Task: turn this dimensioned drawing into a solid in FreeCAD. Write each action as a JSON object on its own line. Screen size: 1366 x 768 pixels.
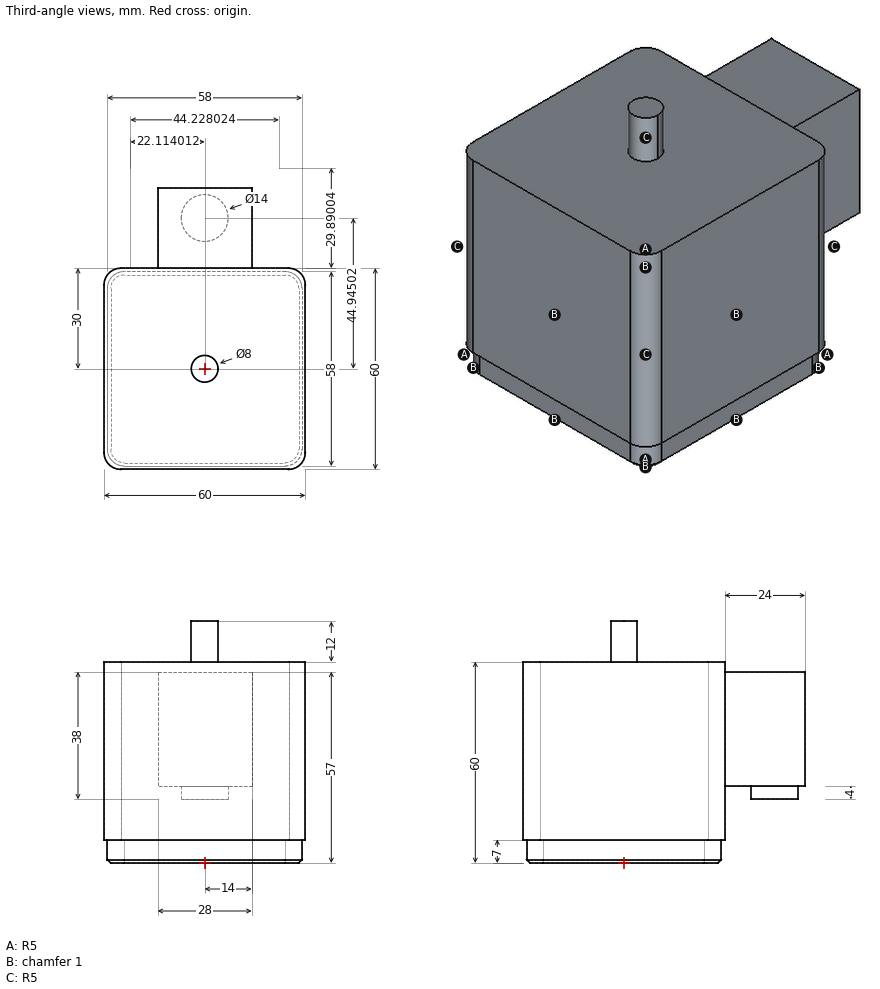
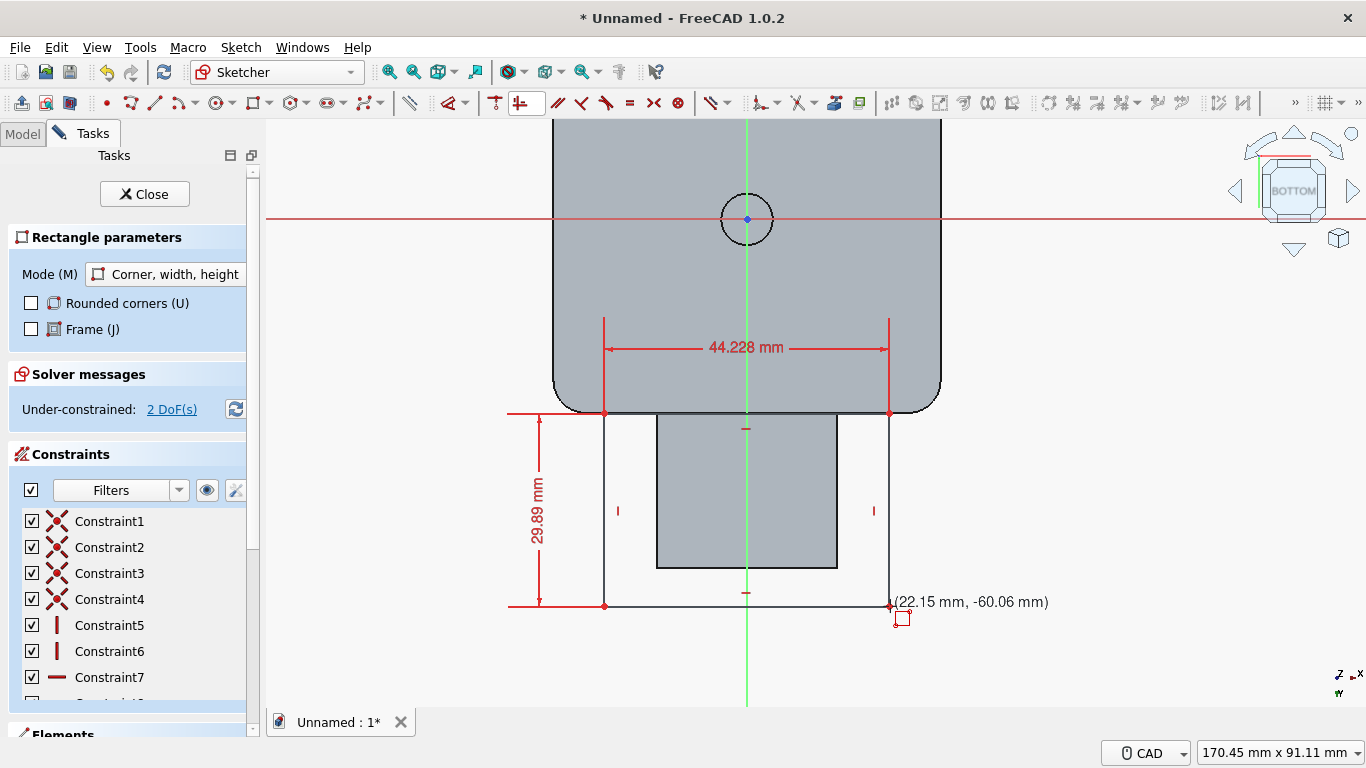
{"action": "key", "text": "g c"}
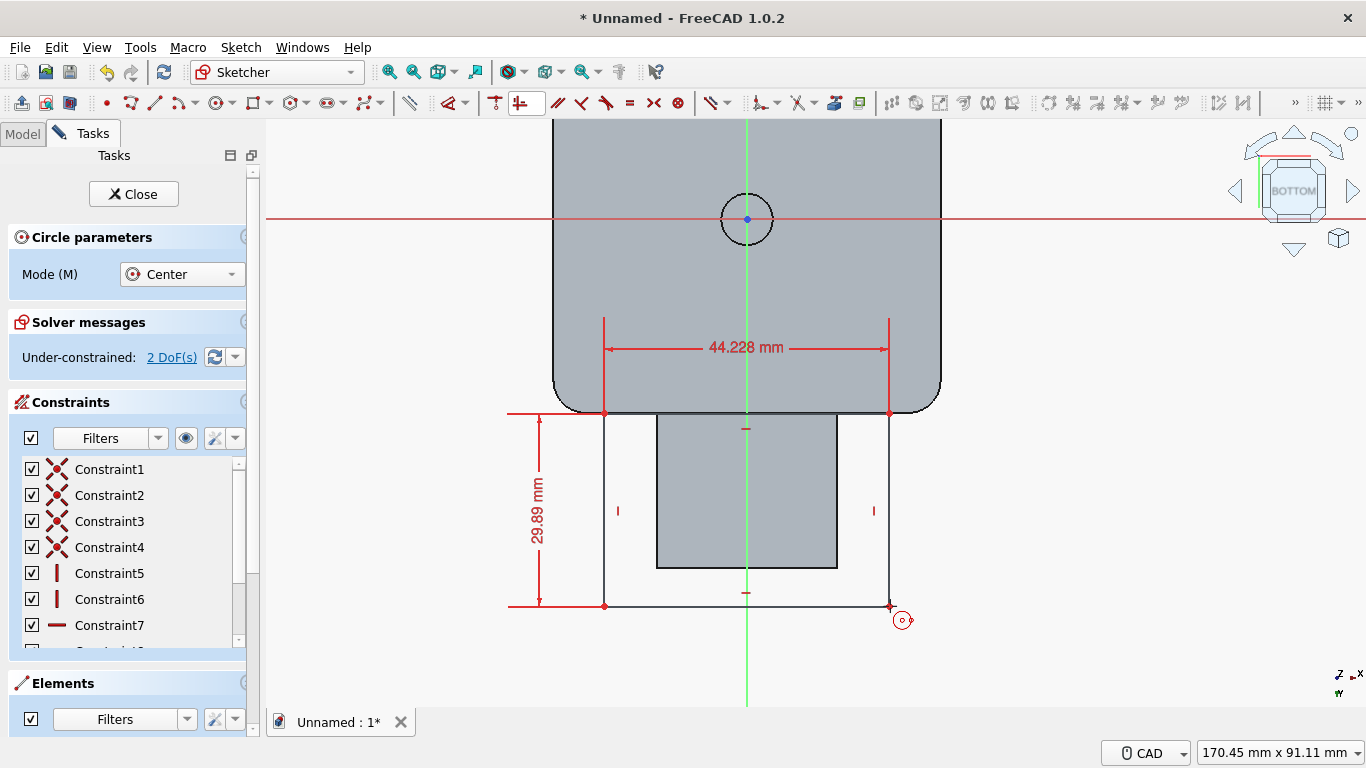
{"action": "left_click", "coordinate": [747, 509]}
{"action": "mouse_move", "coordinate": [779, 478]}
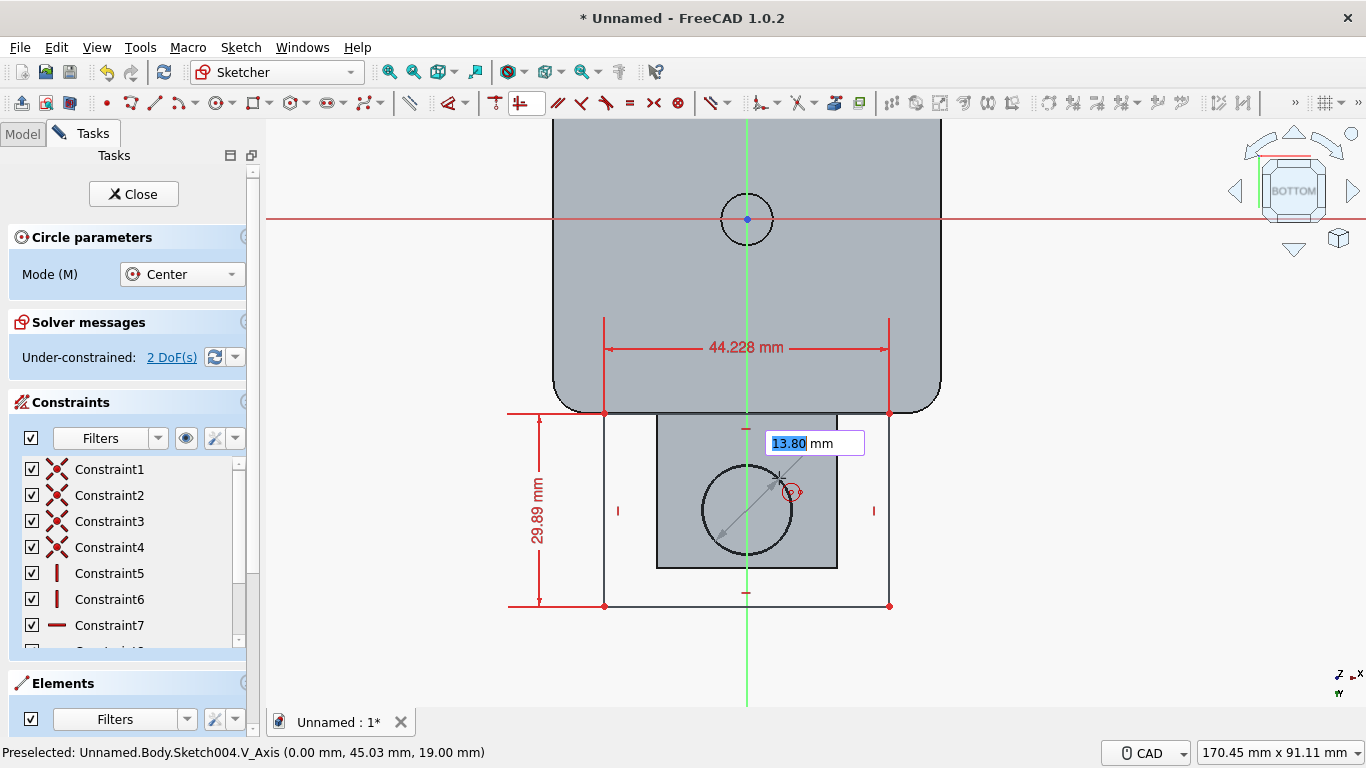
{"action": "type", "text": "14"}
{"action": "key", "text": "Return"}
{"action": "key", "text": "Escape"}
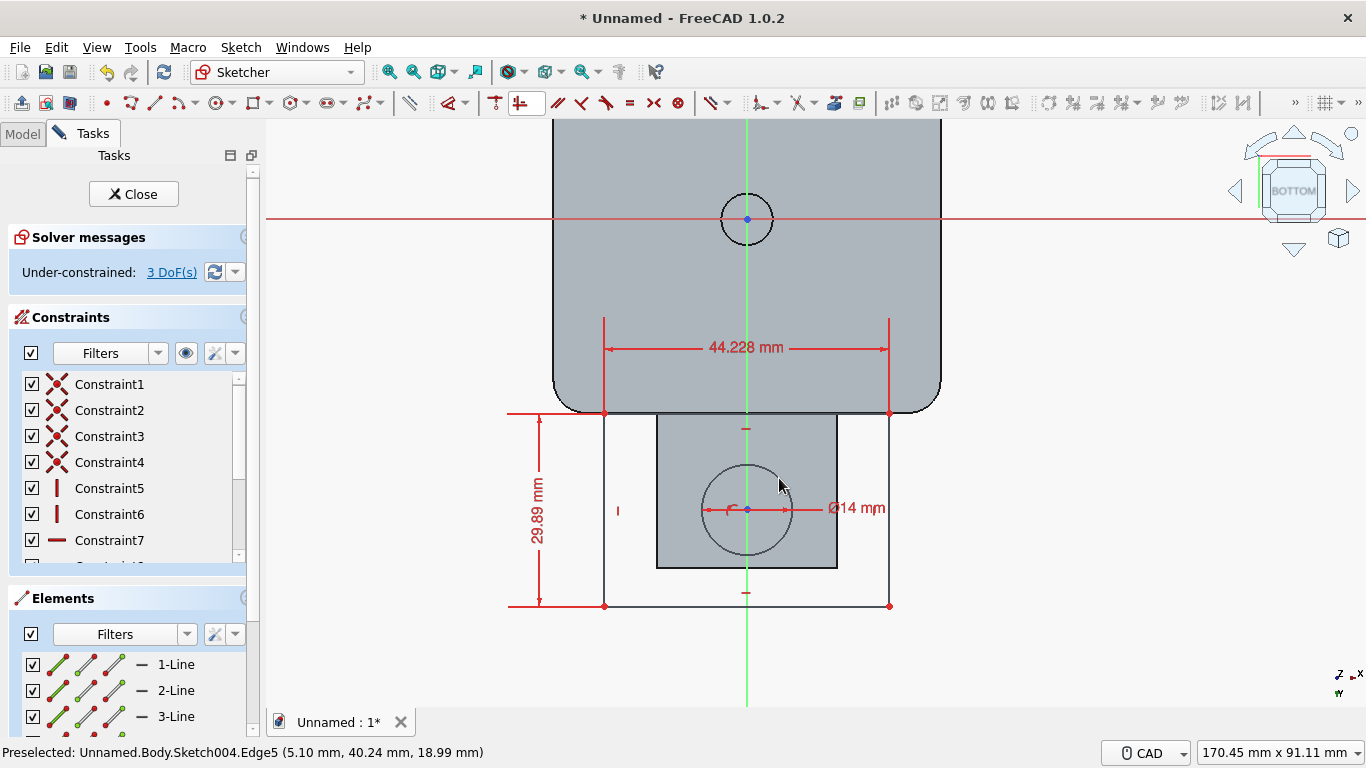
{"action": "key", "text": "d"}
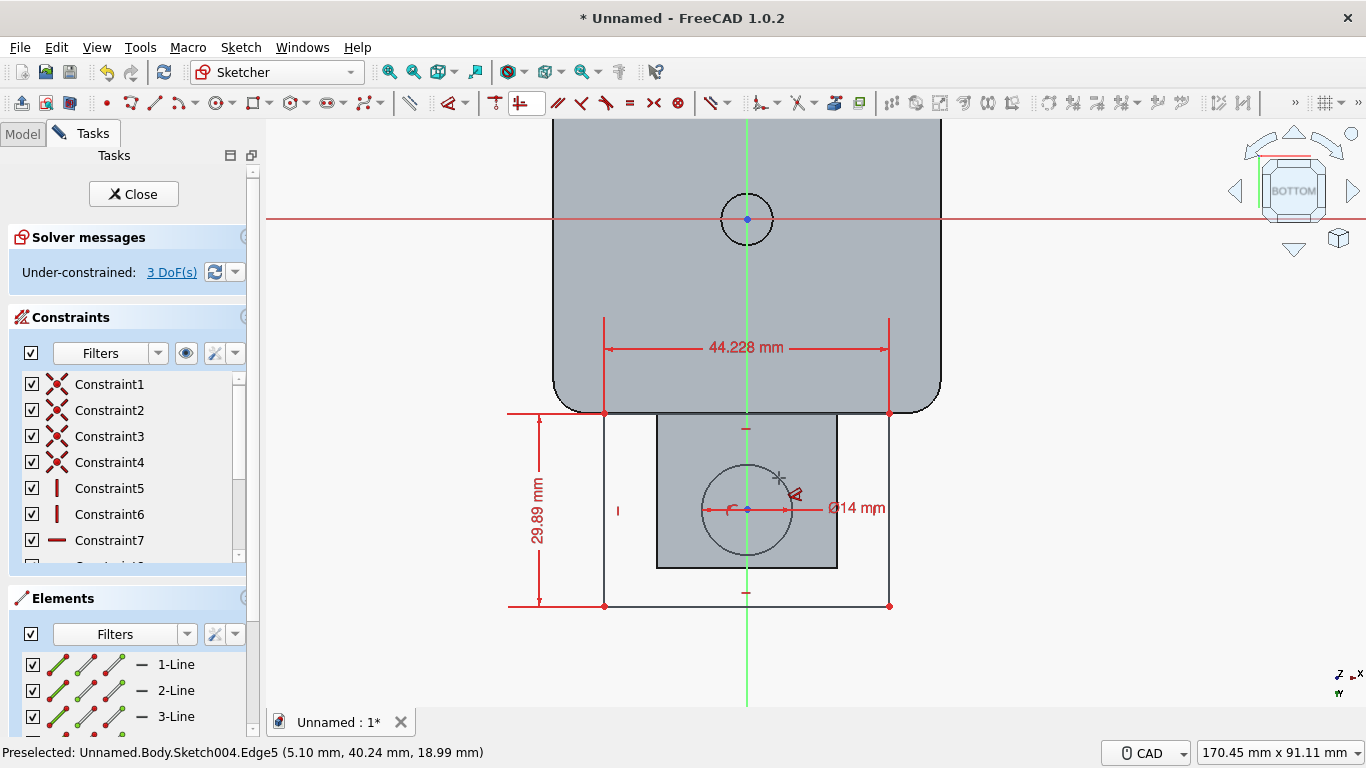
{"action": "left_click", "coordinate": [604, 414]}
{"action": "left_click", "coordinate": [570, 317]}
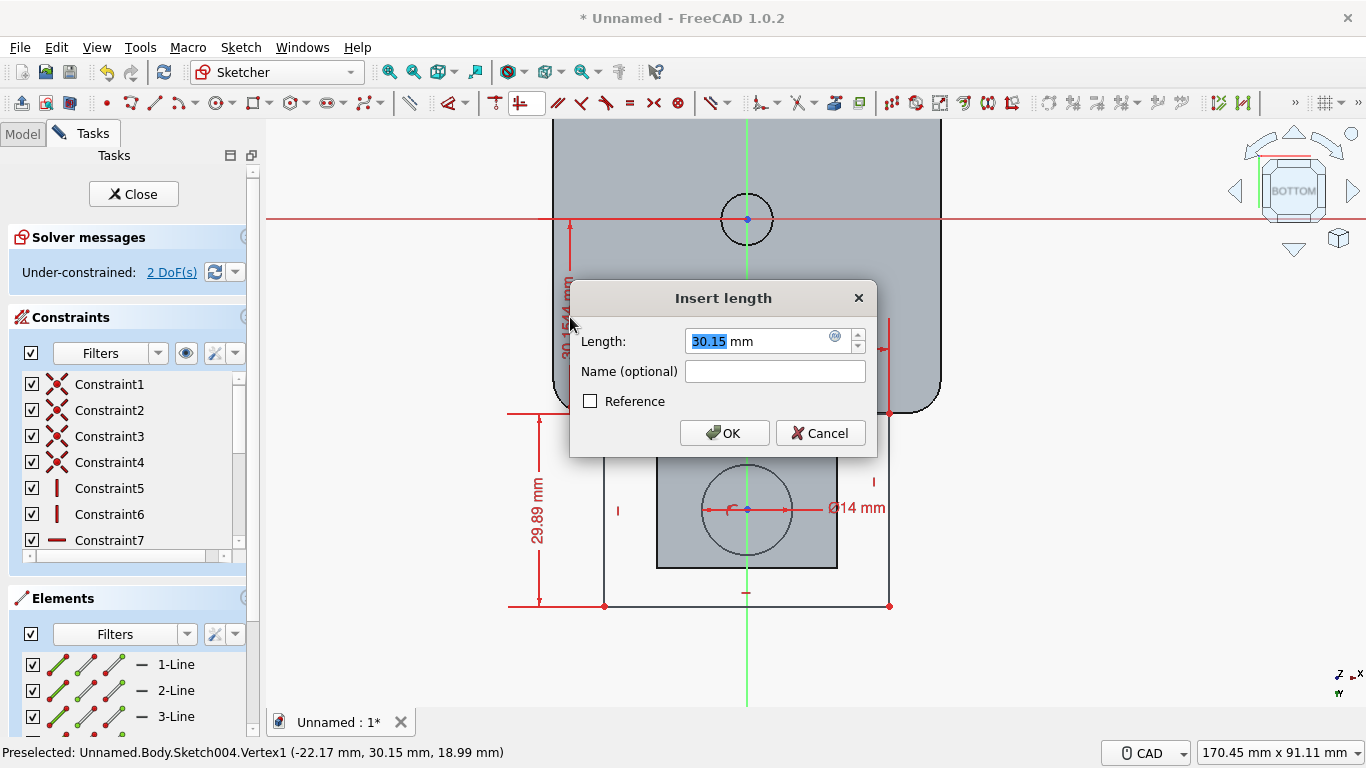
{"action": "type", "text": "30"}
{"action": "key", "text": "Return"}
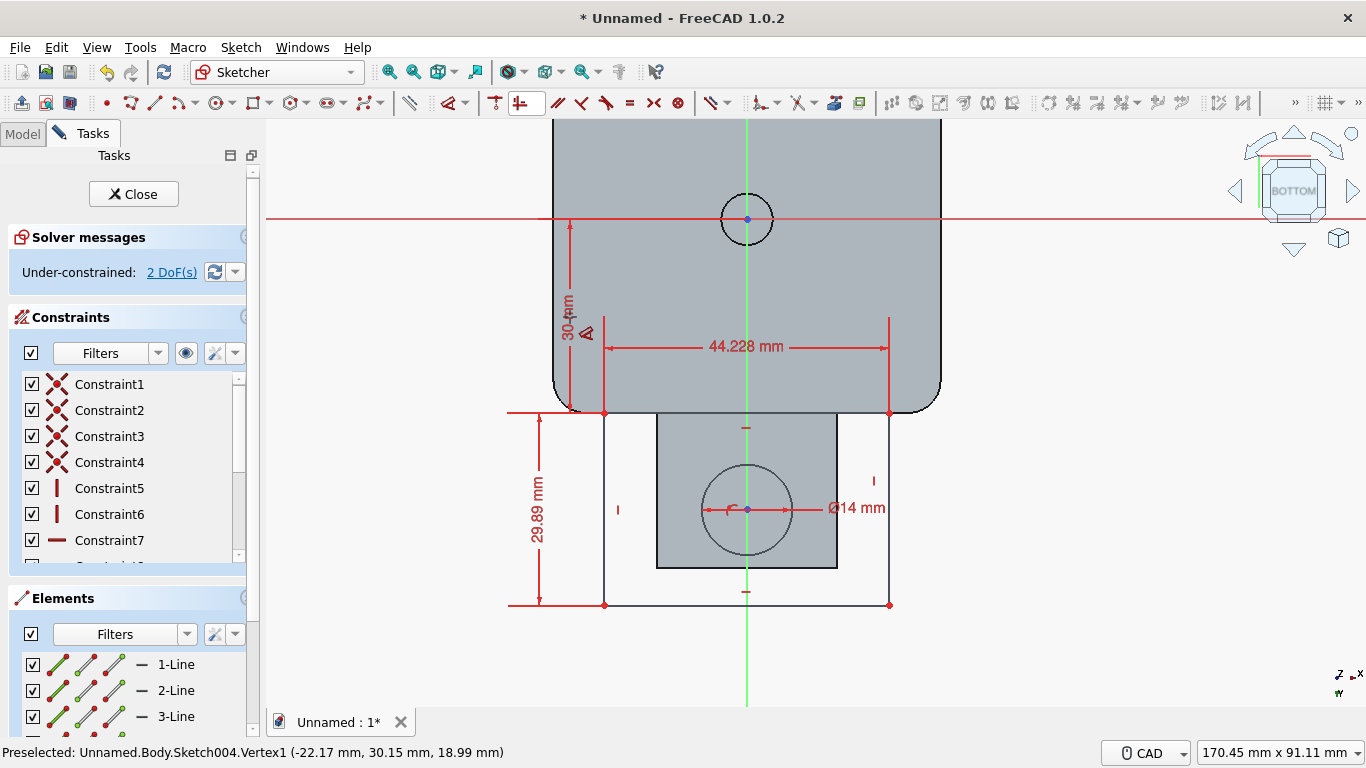
{"action": "left_click", "coordinate": [747, 510]}
{"action": "left_click", "coordinate": [781, 365]}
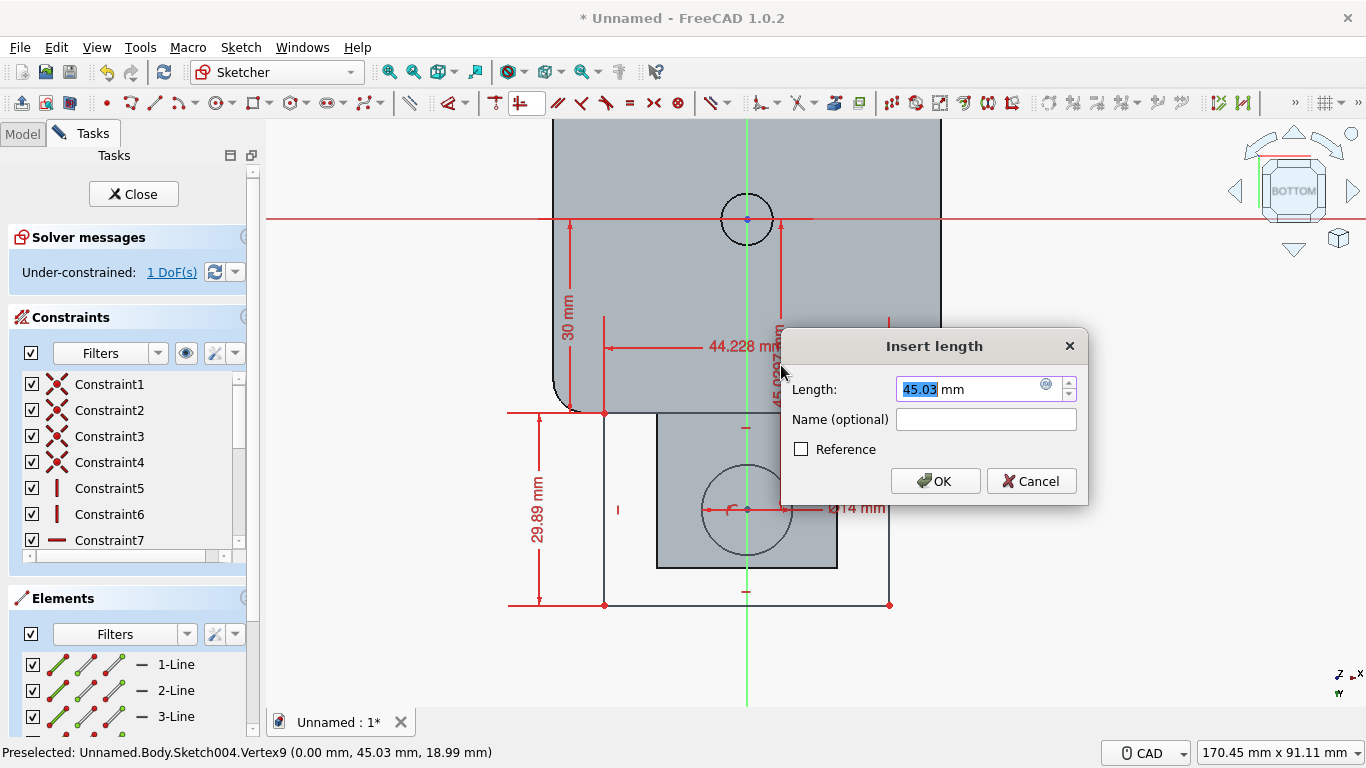
{"action": "type", "text": "44.94502"}
{"action": "key", "text": "Return"}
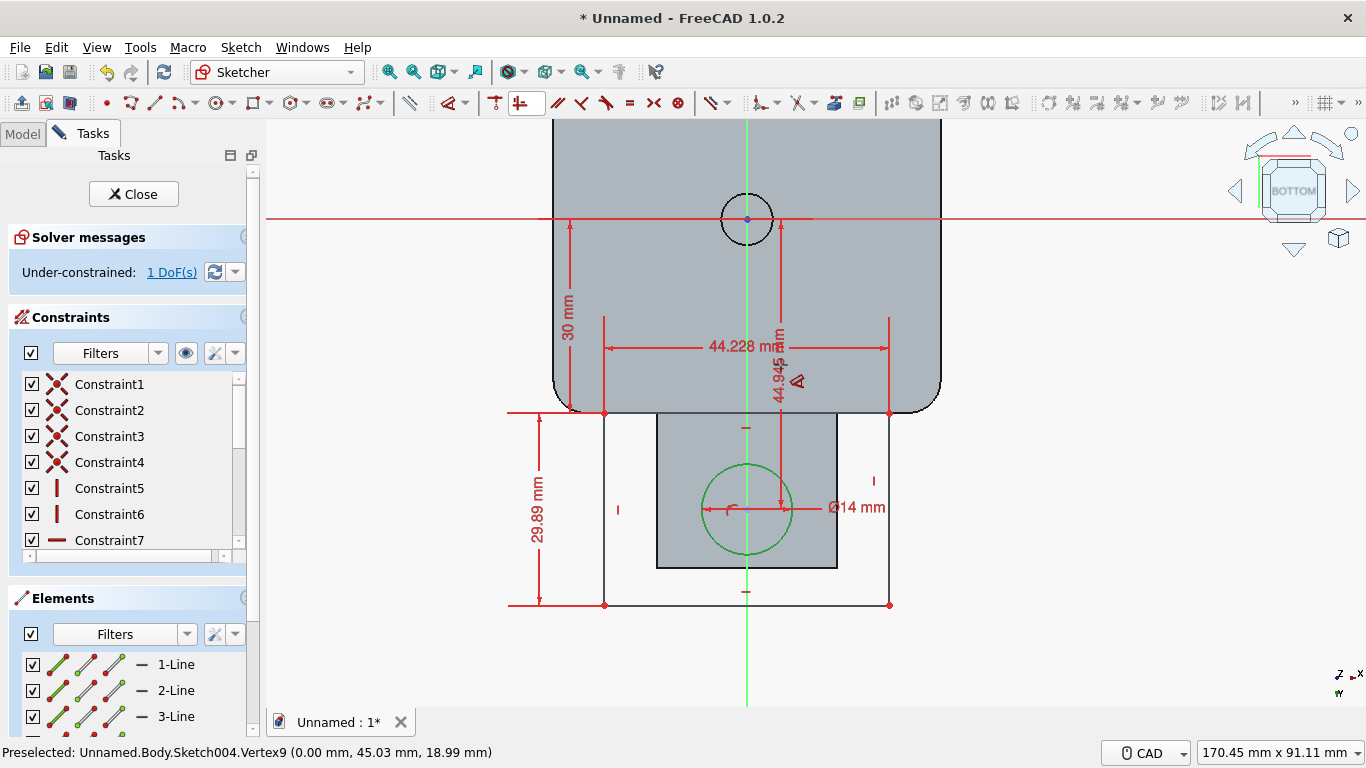
{"action": "left_click", "coordinate": [604, 413]}
{"action": "left_click", "coordinate": [676, 185]}